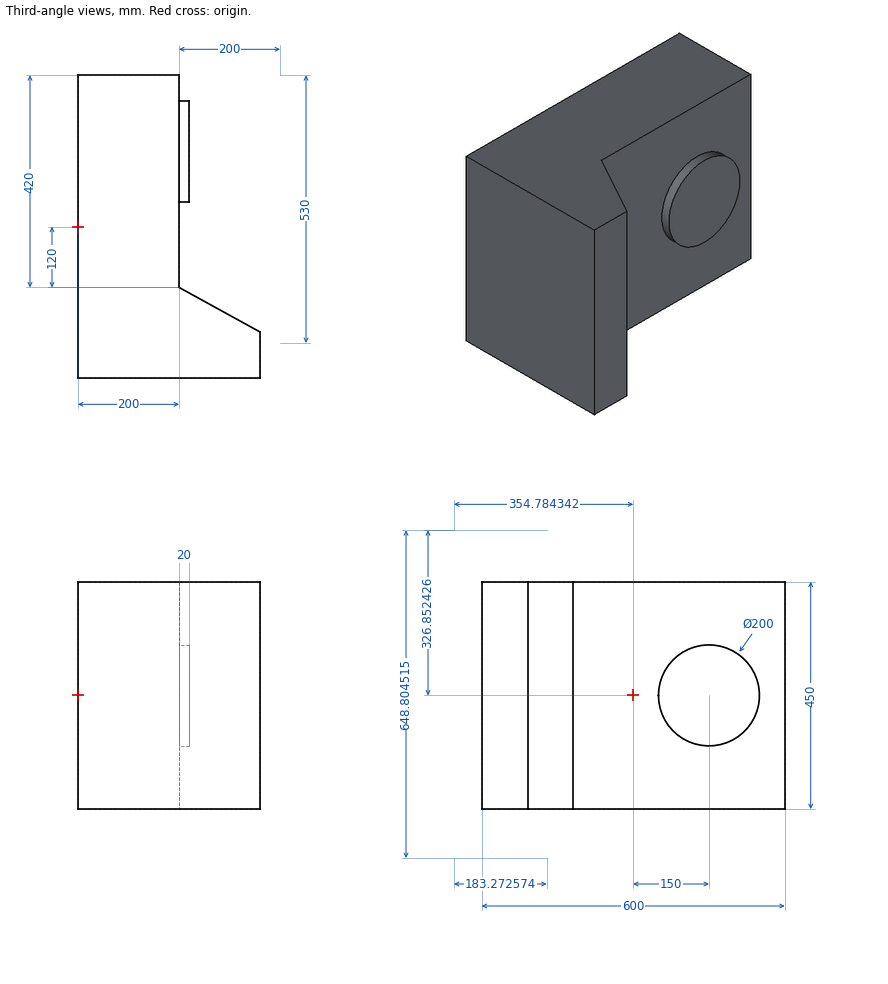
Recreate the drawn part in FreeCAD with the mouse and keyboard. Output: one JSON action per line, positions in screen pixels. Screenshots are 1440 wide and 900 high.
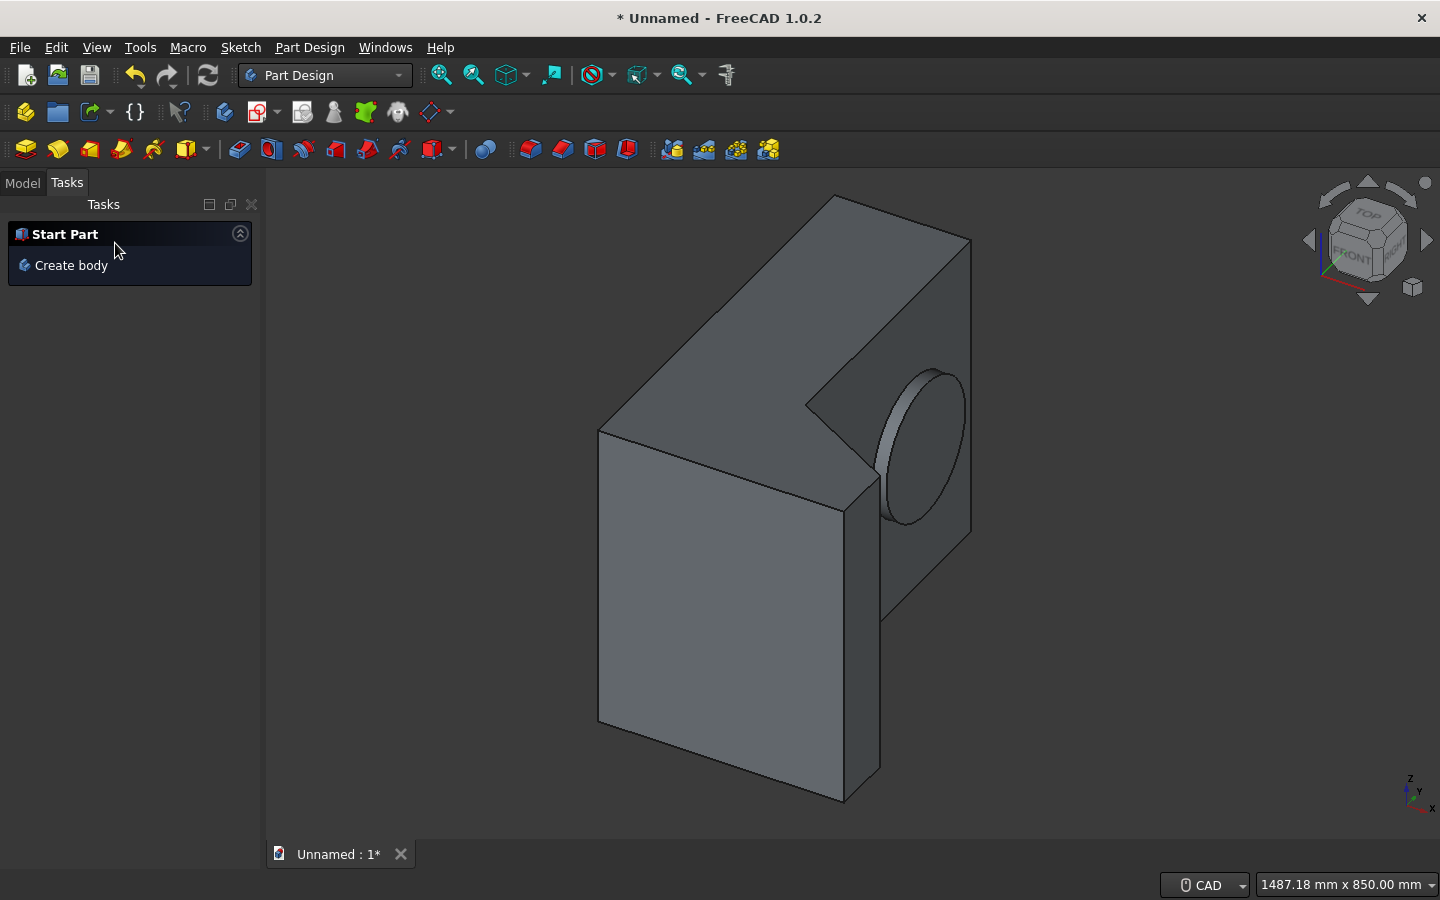
{"action": "key", "text": "0"}